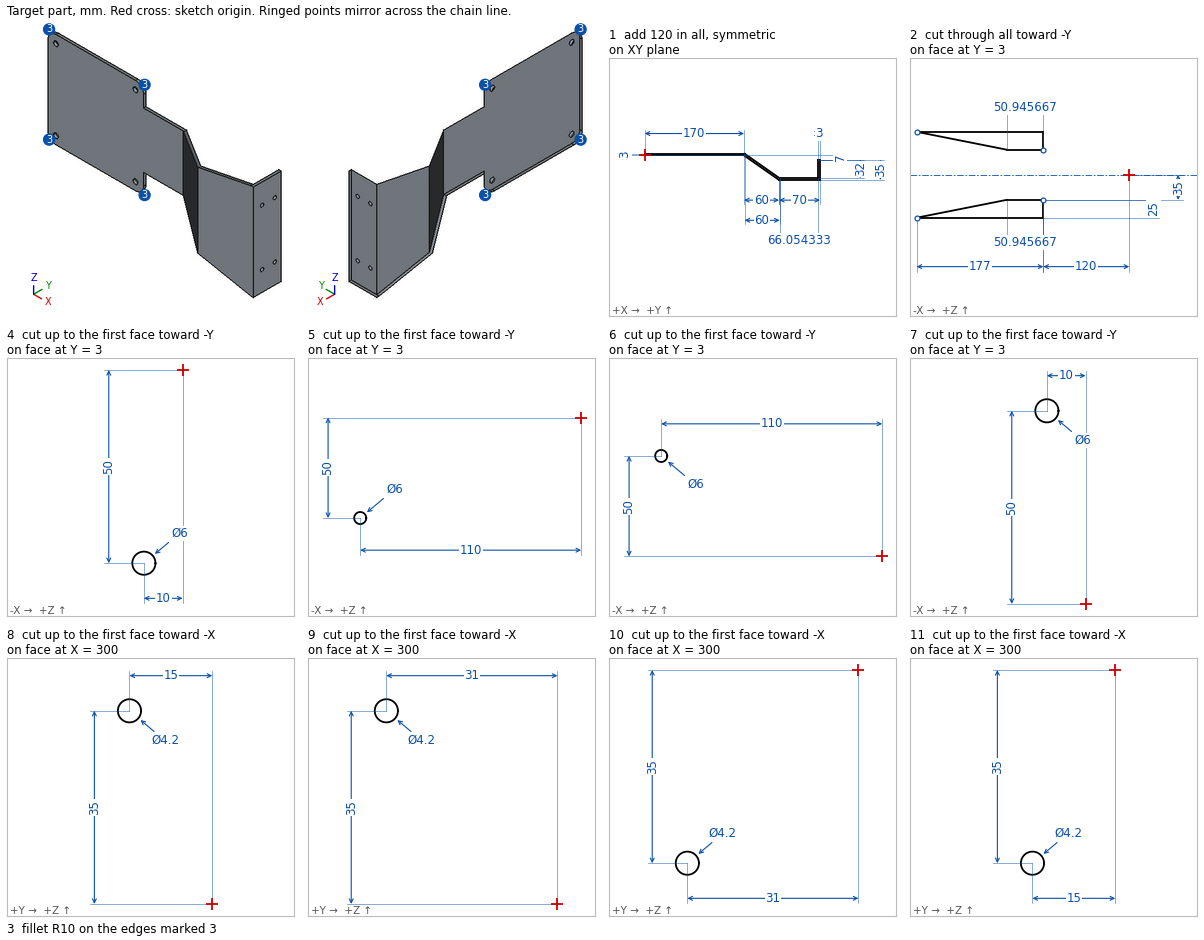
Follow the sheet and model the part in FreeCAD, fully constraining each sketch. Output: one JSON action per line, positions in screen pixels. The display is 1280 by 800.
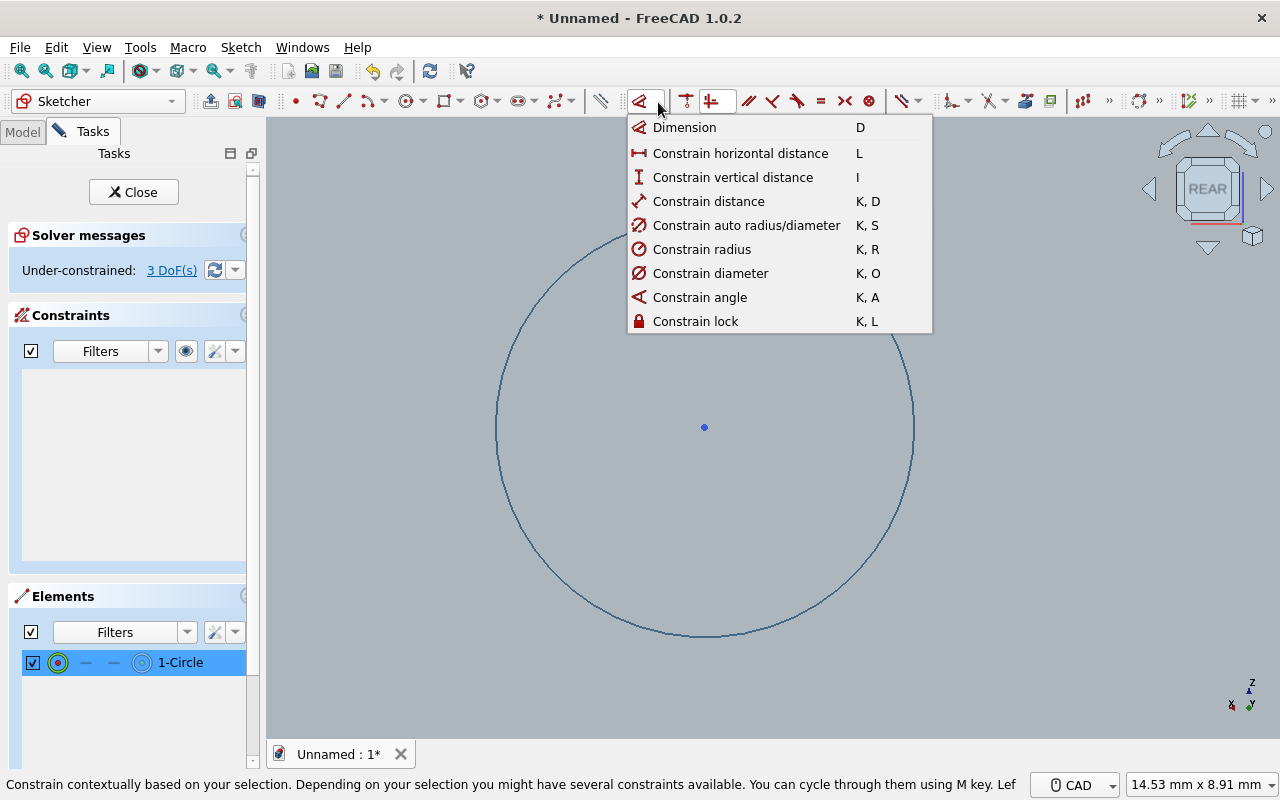
{"action": "left_click", "coordinate": [780, 273]}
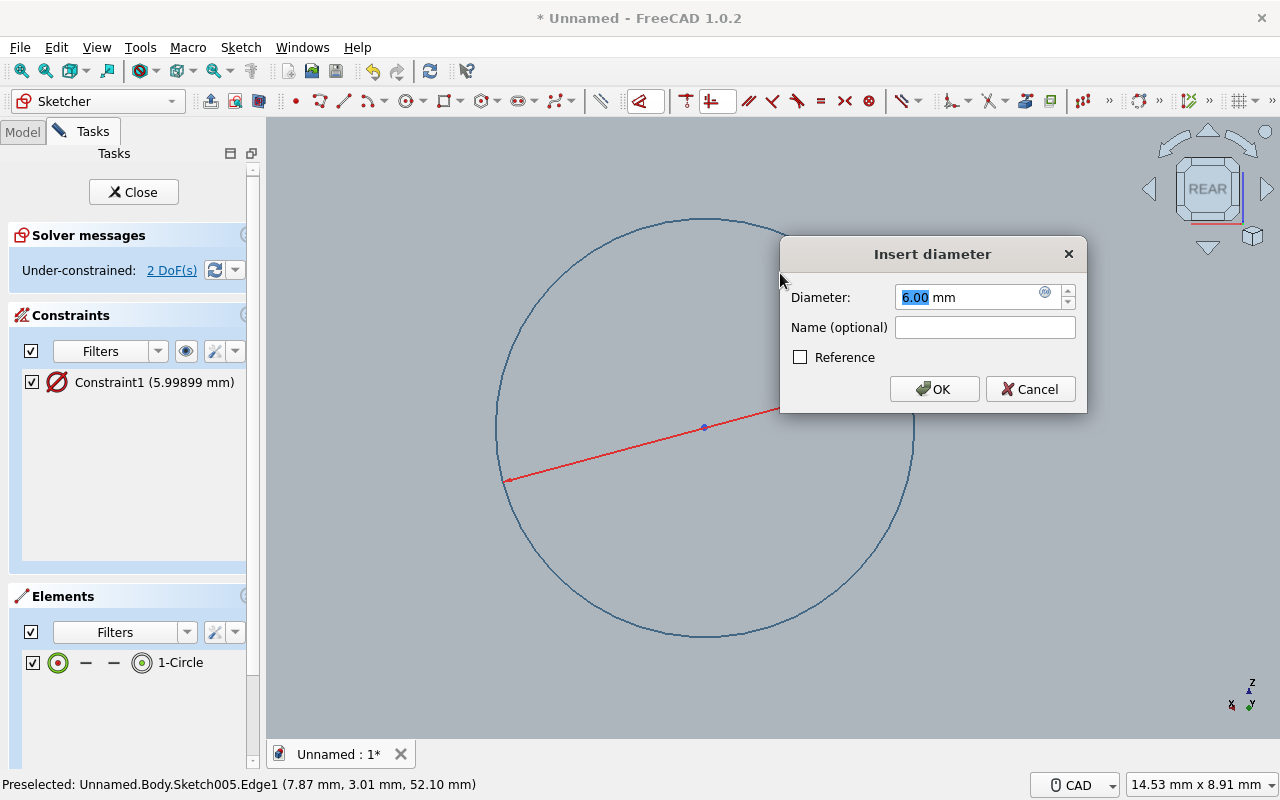
{"action": "type", "text": "6"}
{"action": "key", "text": "Return"}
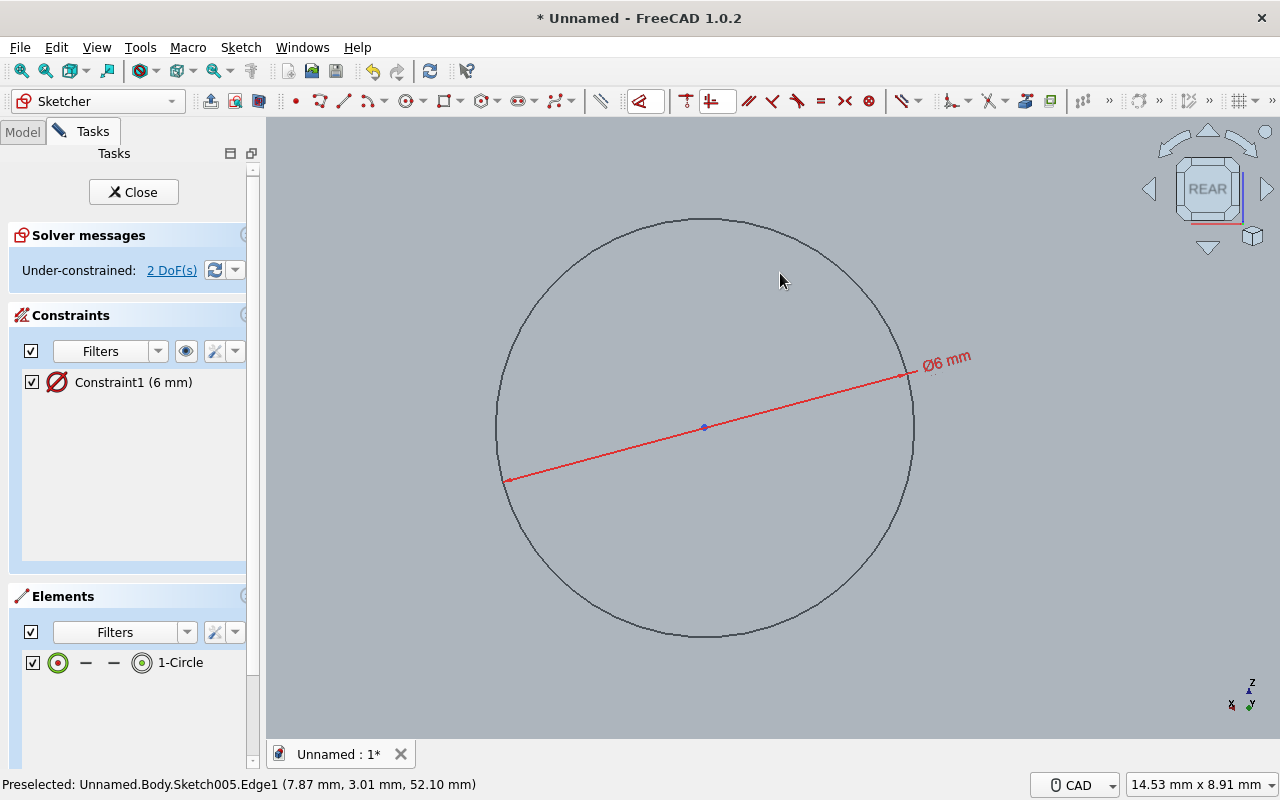
{"action": "left_click", "coordinate": [705, 428]}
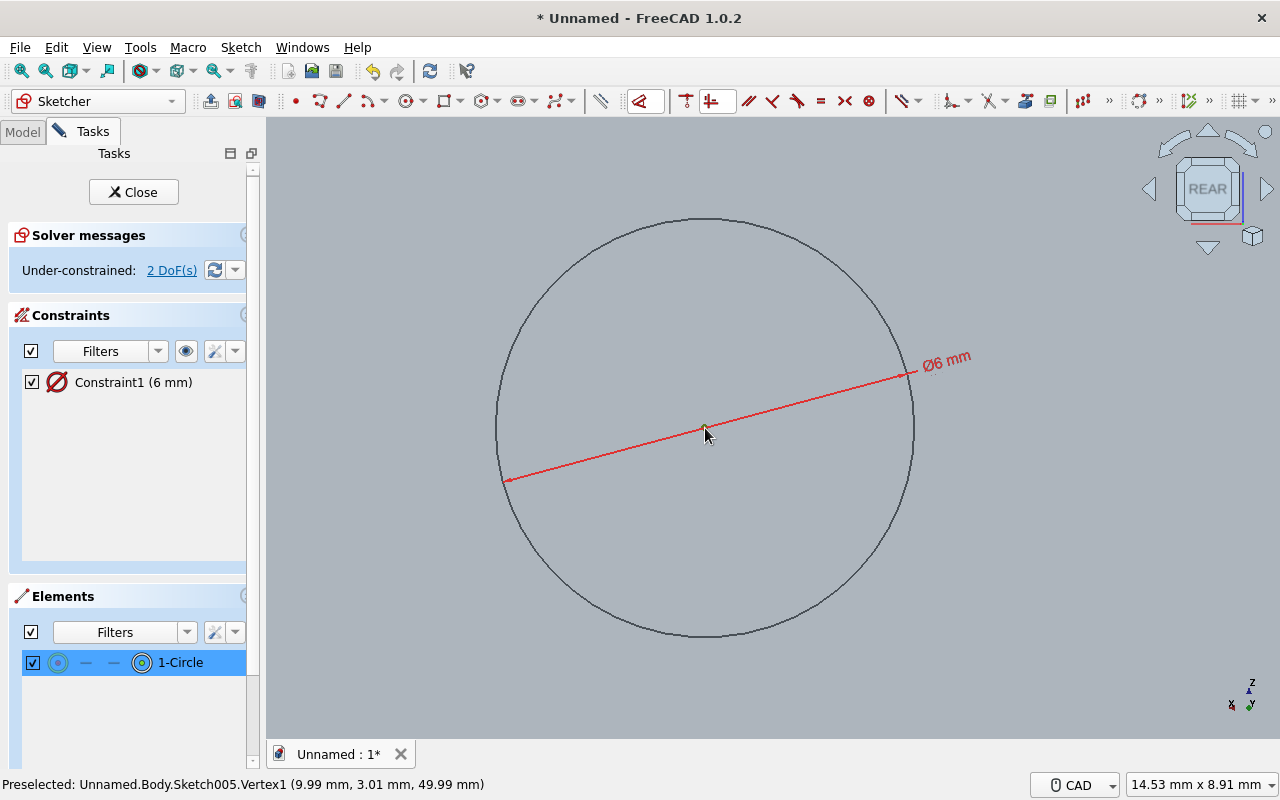
{"action": "left_click", "coordinate": [658, 102]}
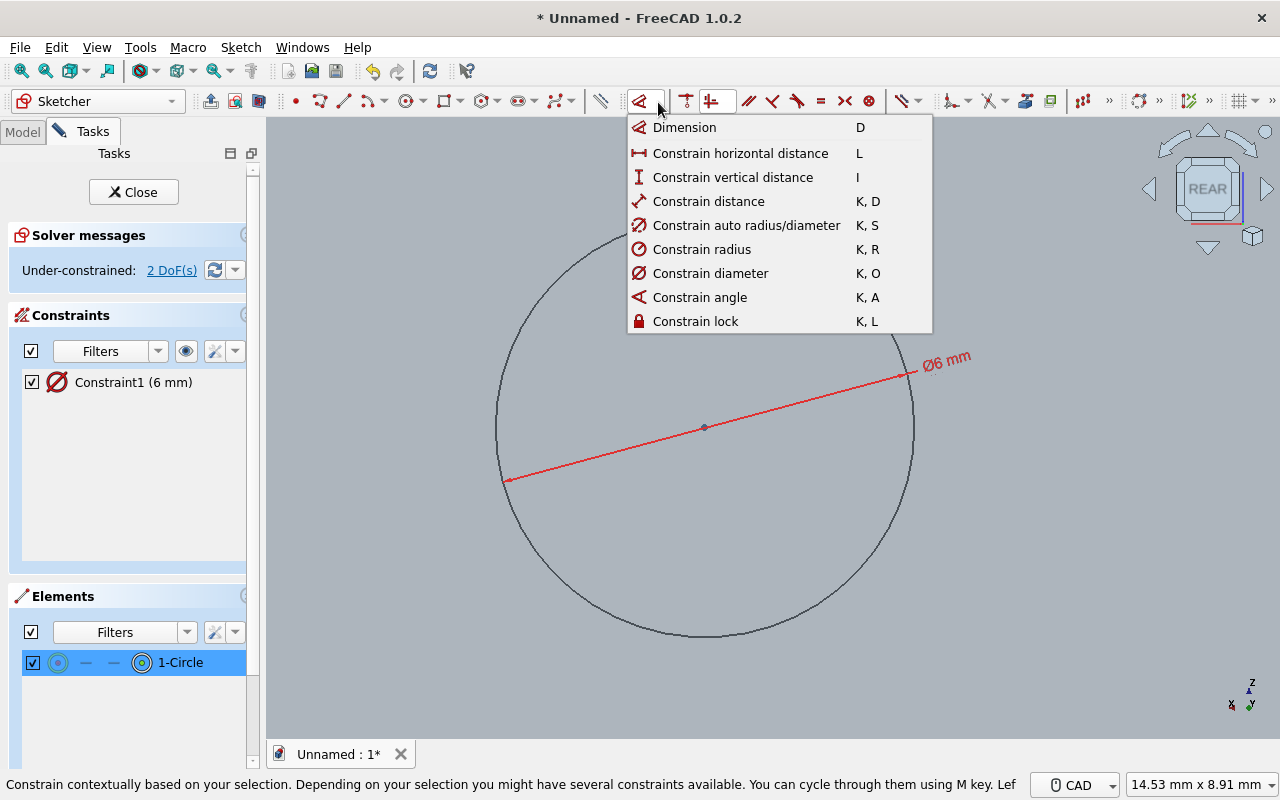
{"action": "left_click", "coordinate": [780, 153]}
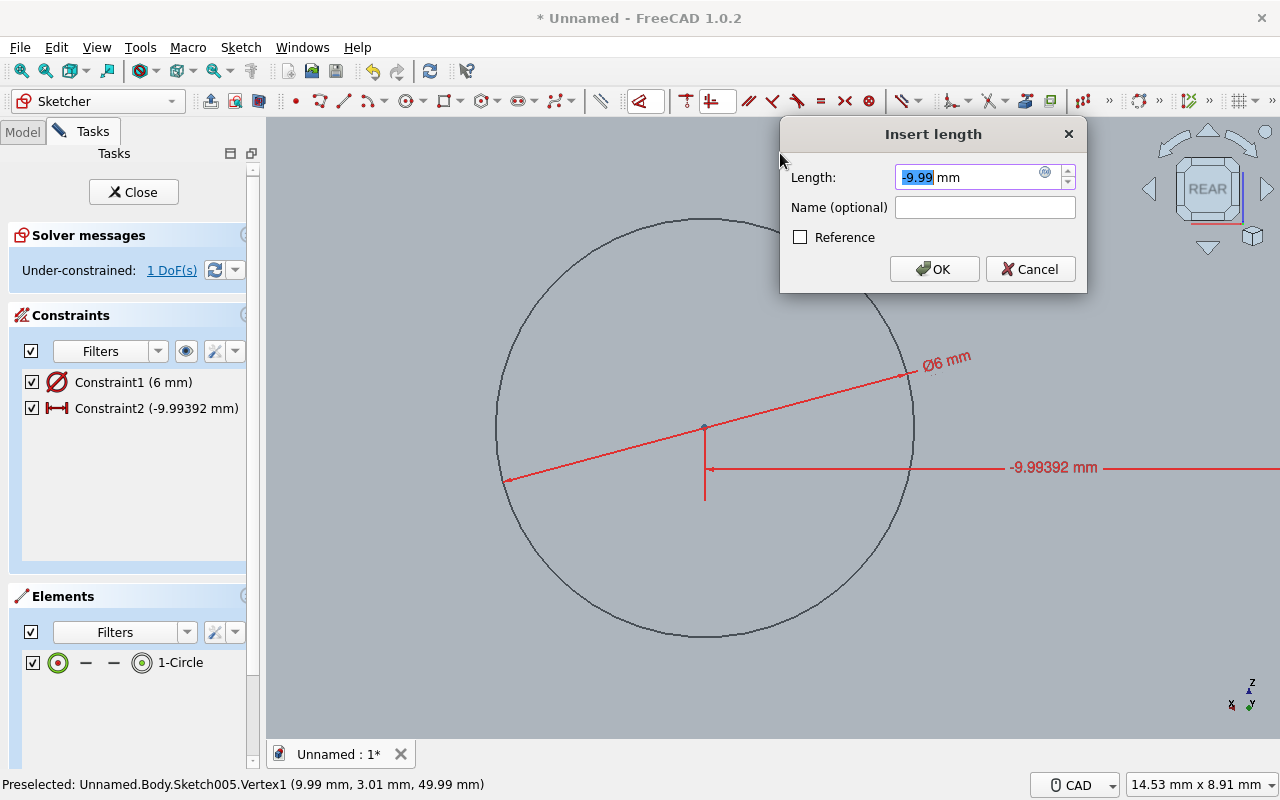
{"action": "type", "text": "-10"}
{"action": "key", "text": "Return"}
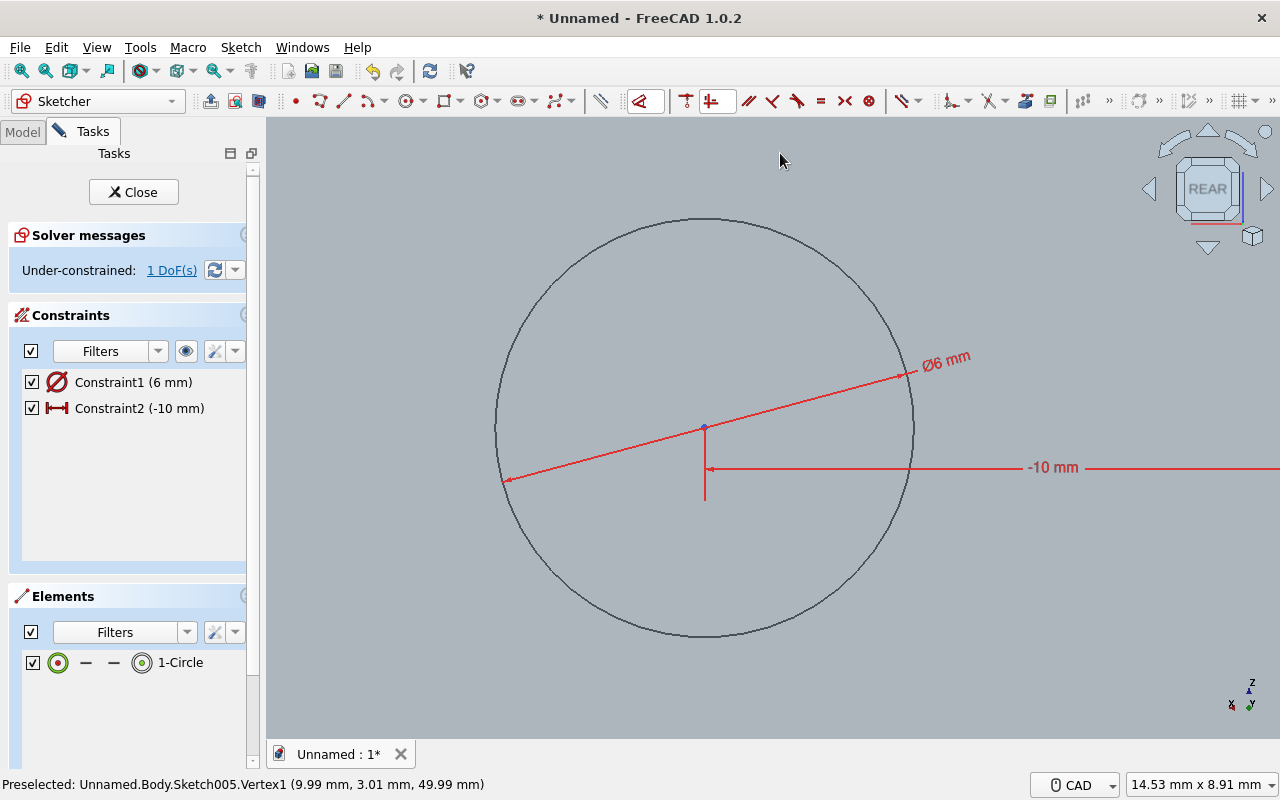
{"action": "left_click", "coordinate": [705, 428]}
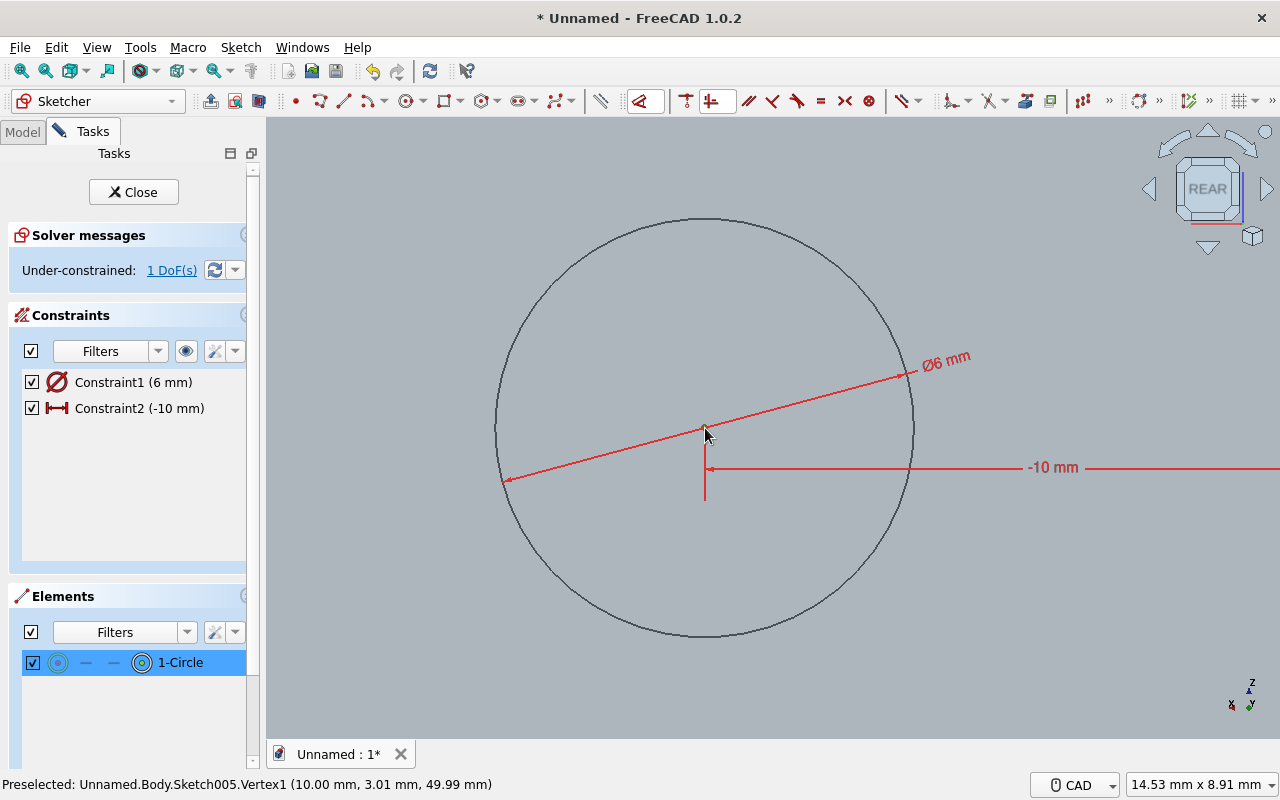
{"action": "left_click", "coordinate": [658, 102]}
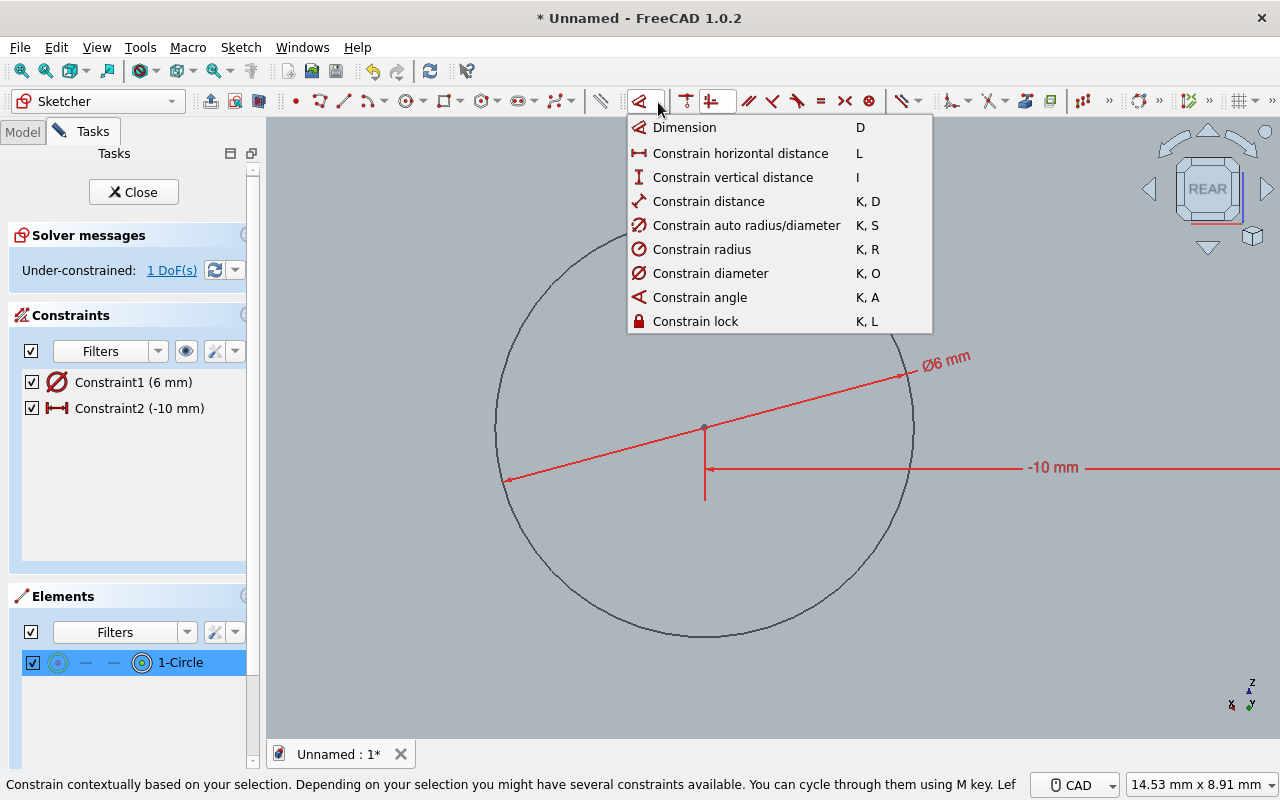
{"action": "left_click", "coordinate": [780, 177]}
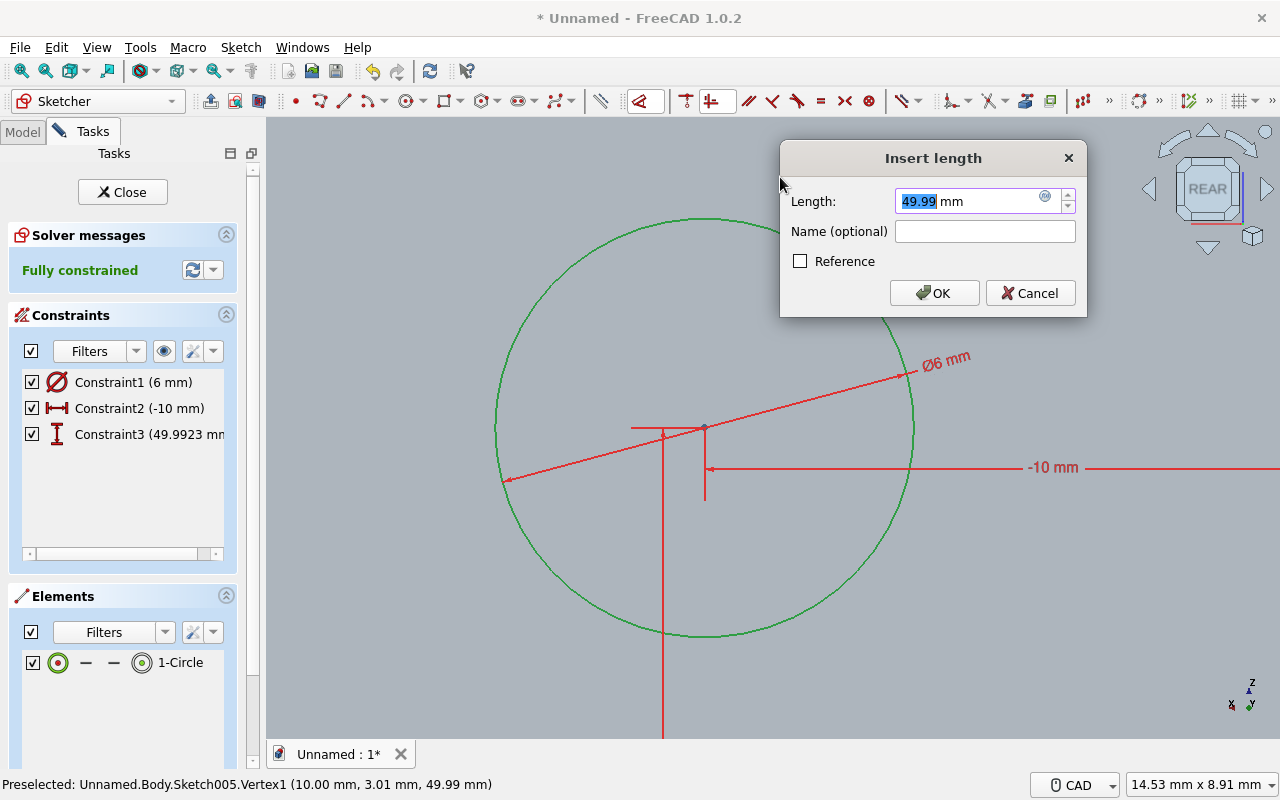
{"action": "type", "text": "50"}
{"action": "key", "text": "Return"}